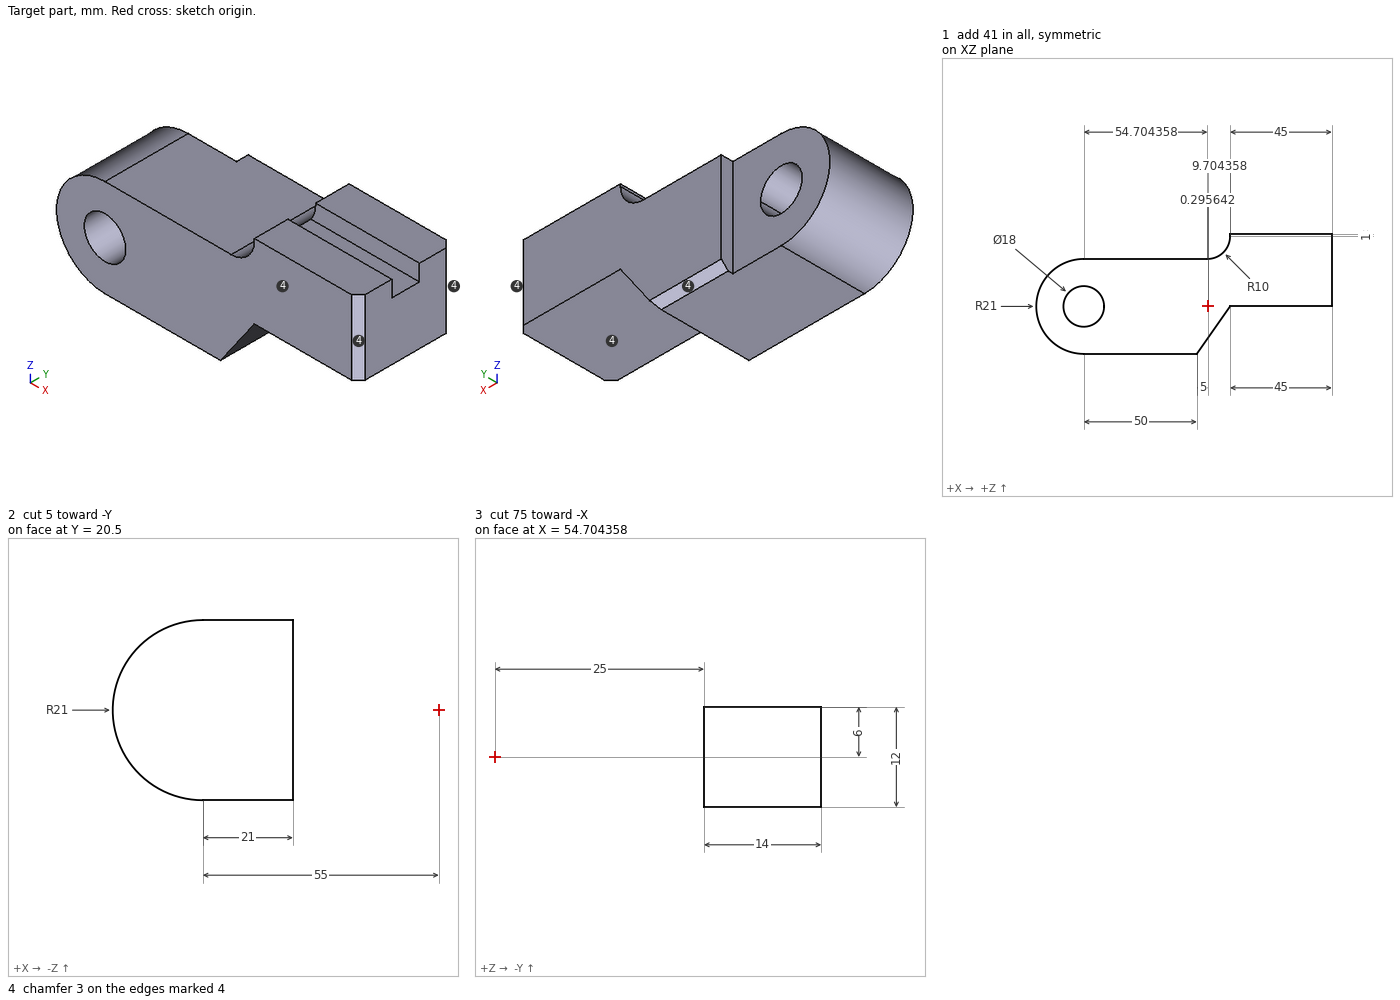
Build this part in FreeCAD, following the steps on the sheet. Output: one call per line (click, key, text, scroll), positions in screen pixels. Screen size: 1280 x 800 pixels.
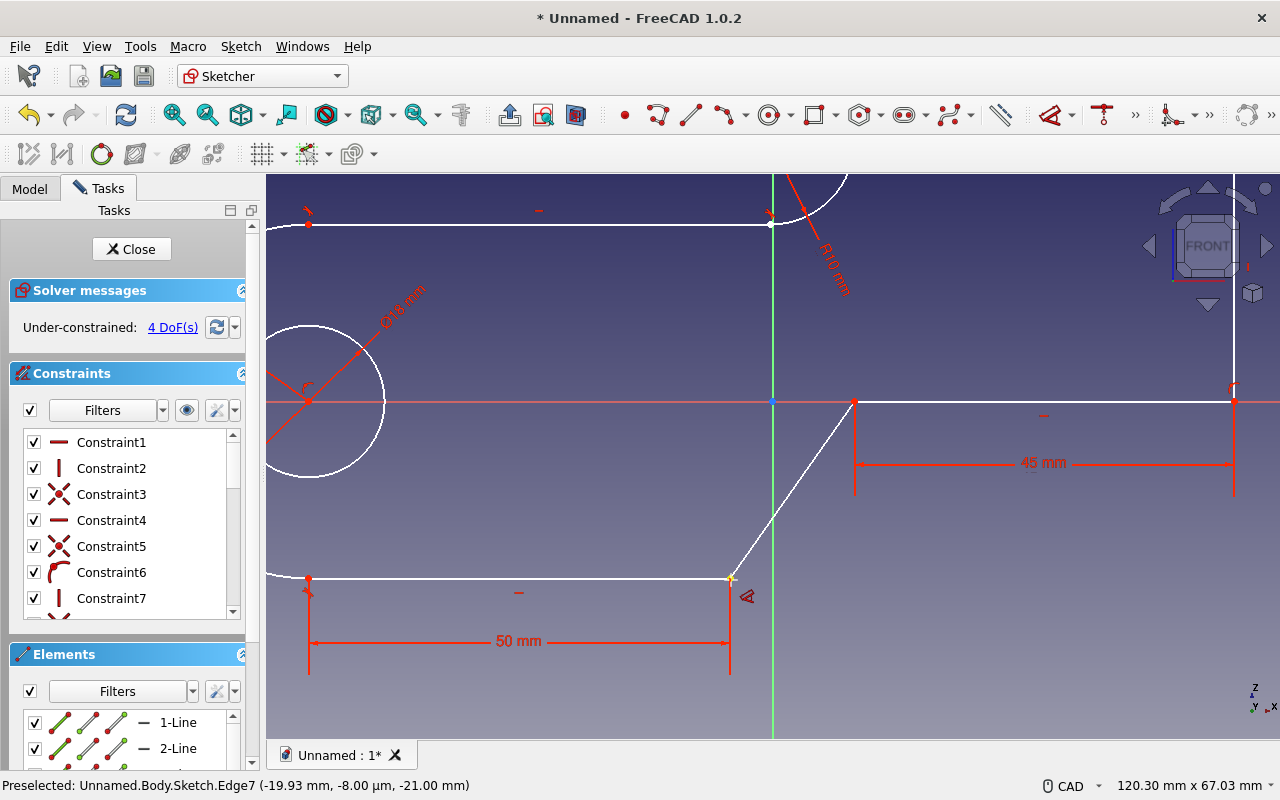
click(730, 579)
click(752, 613)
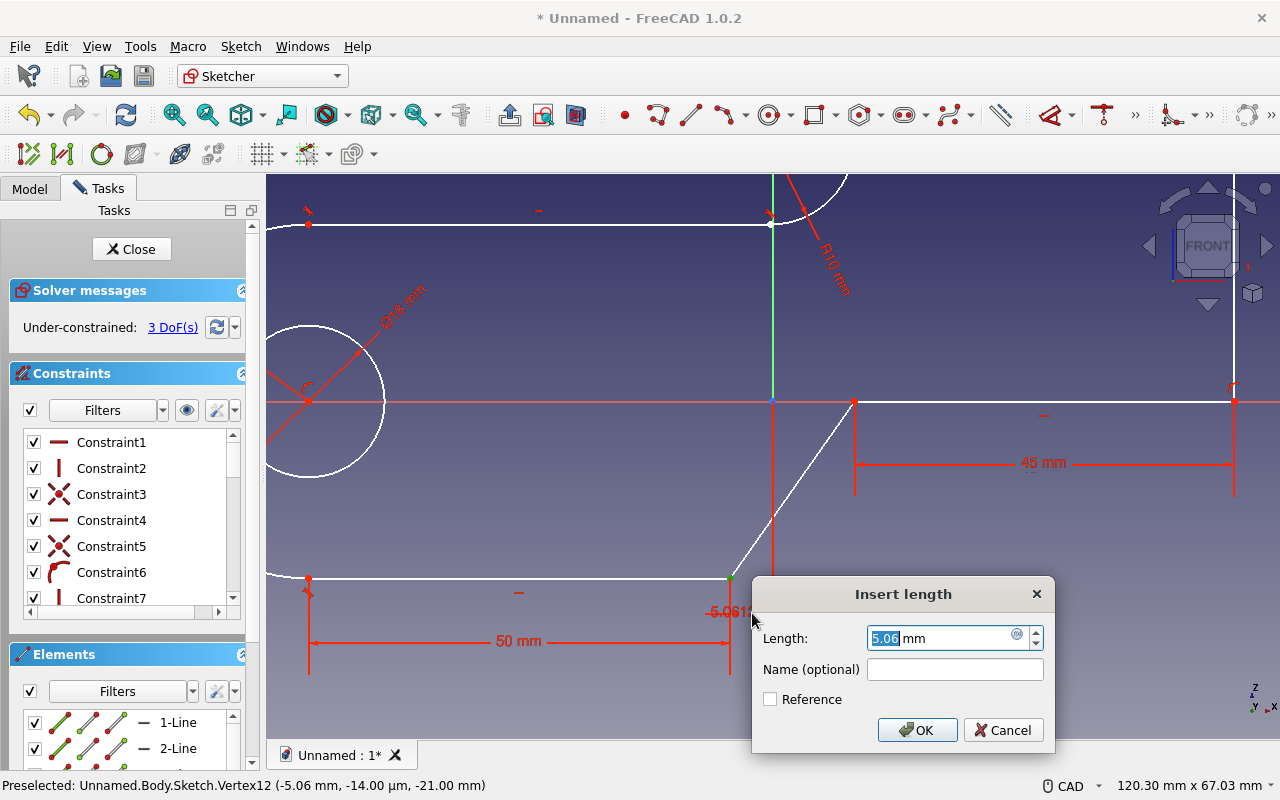
text(5)
key(Return)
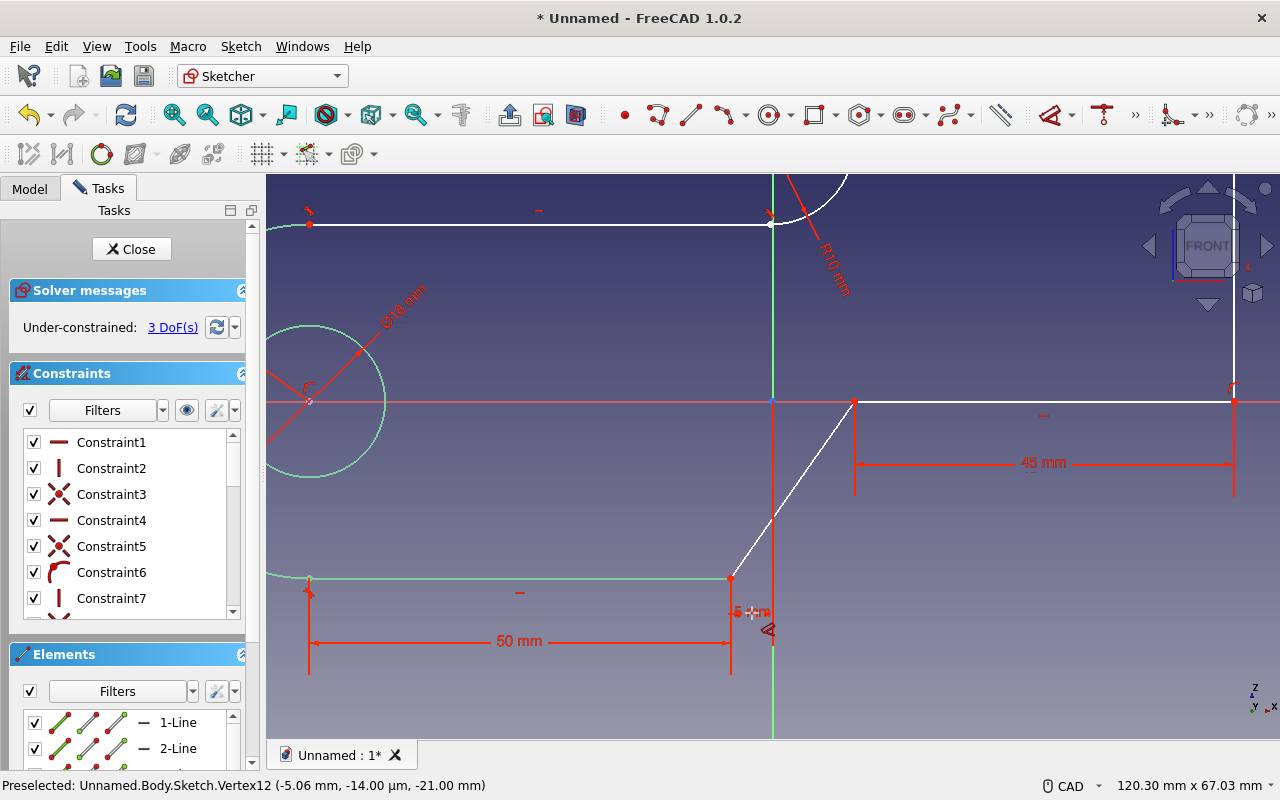
click(448, 225)
click(540, 259)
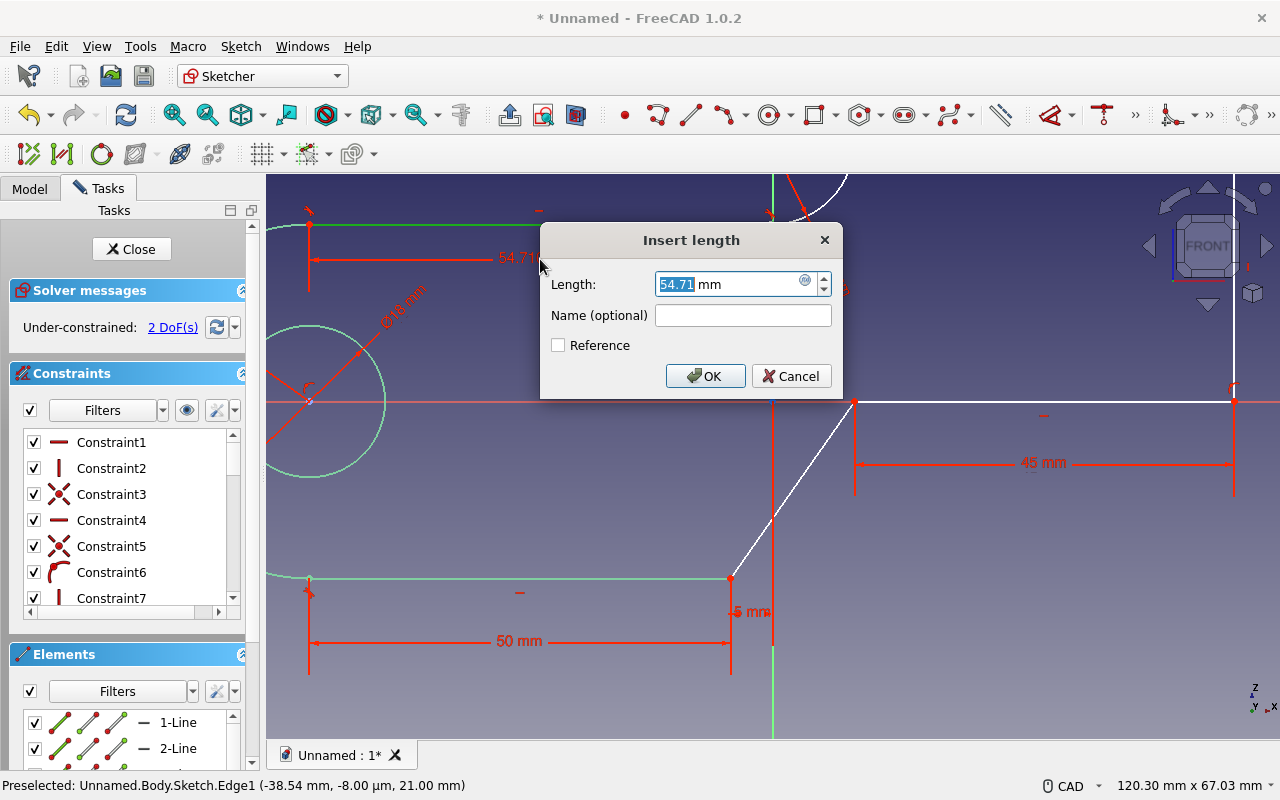
text(54.704358)
key(Return)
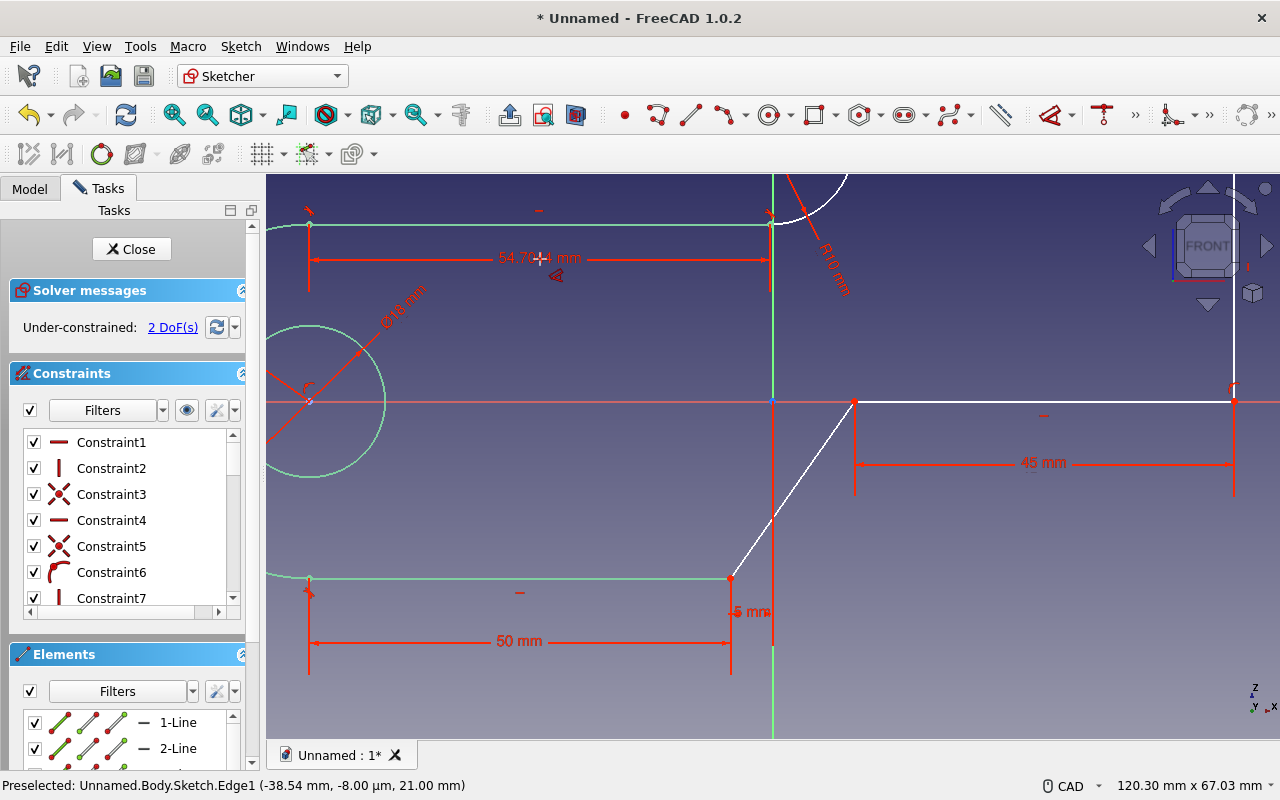
scroll(730, 580, down, 3)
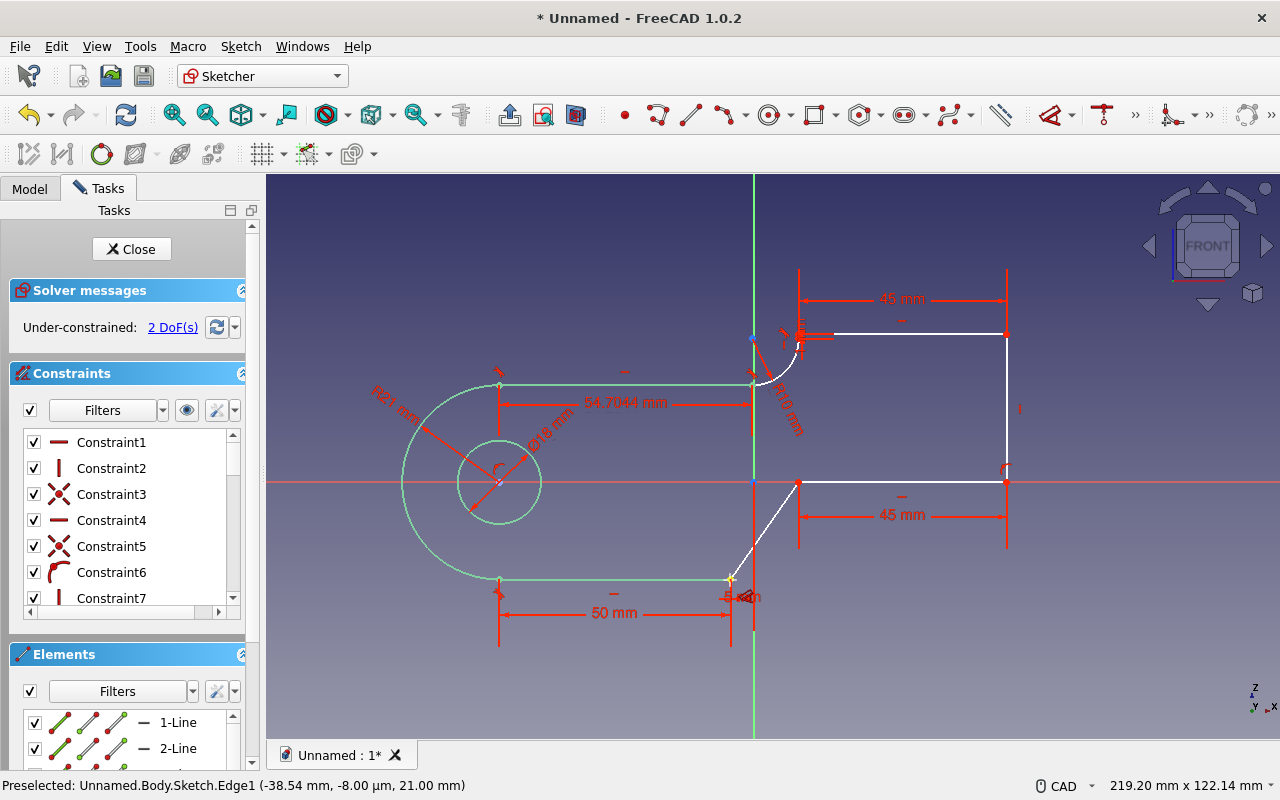
scroll(799, 339, up, 5)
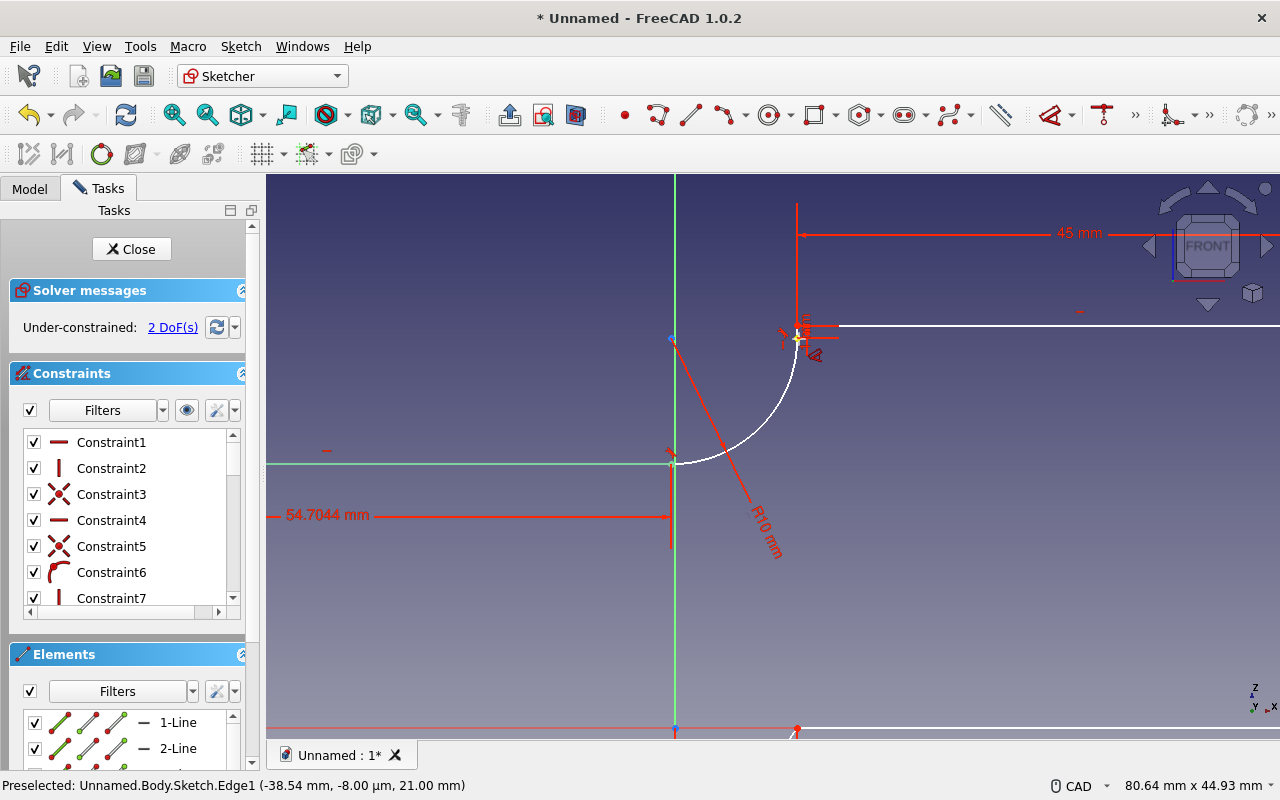
click(797, 338)
click(736, 304)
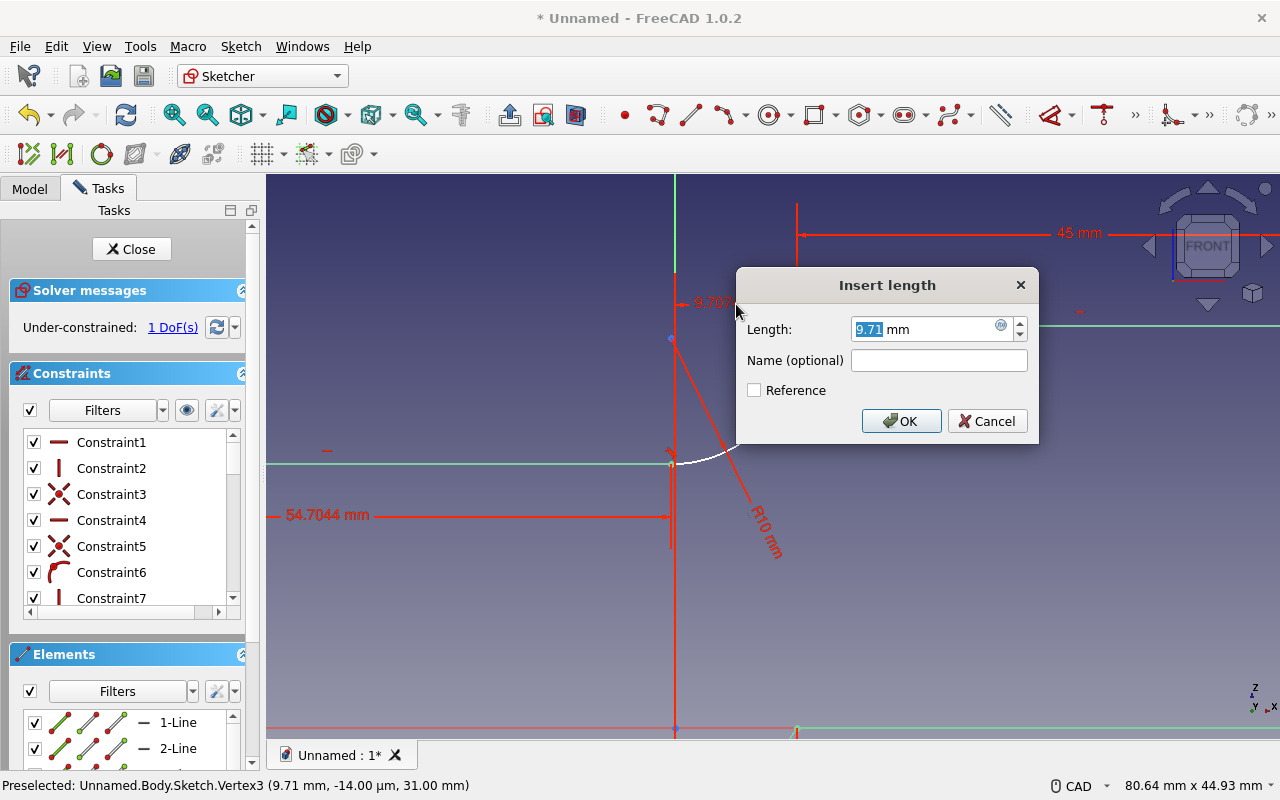
text(9.704358)
key(Return)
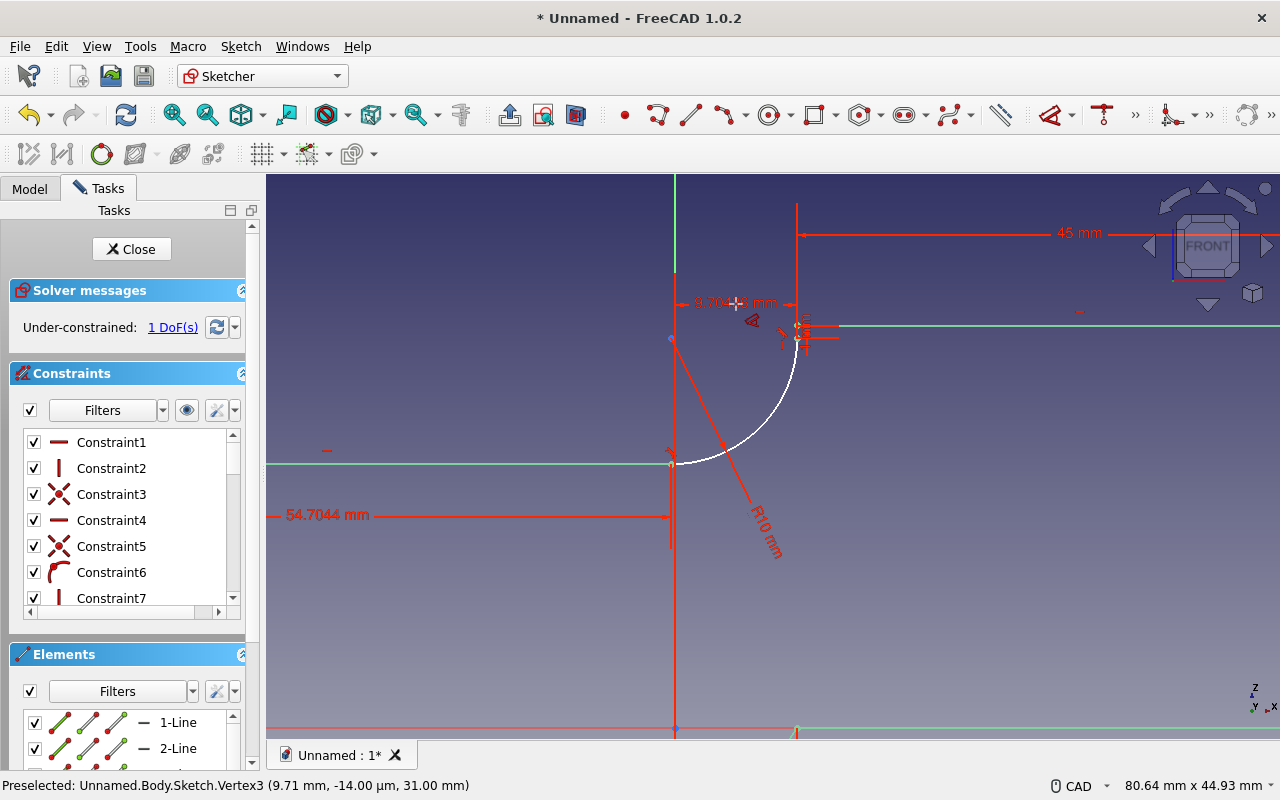
scroll(671, 464, up, 12)